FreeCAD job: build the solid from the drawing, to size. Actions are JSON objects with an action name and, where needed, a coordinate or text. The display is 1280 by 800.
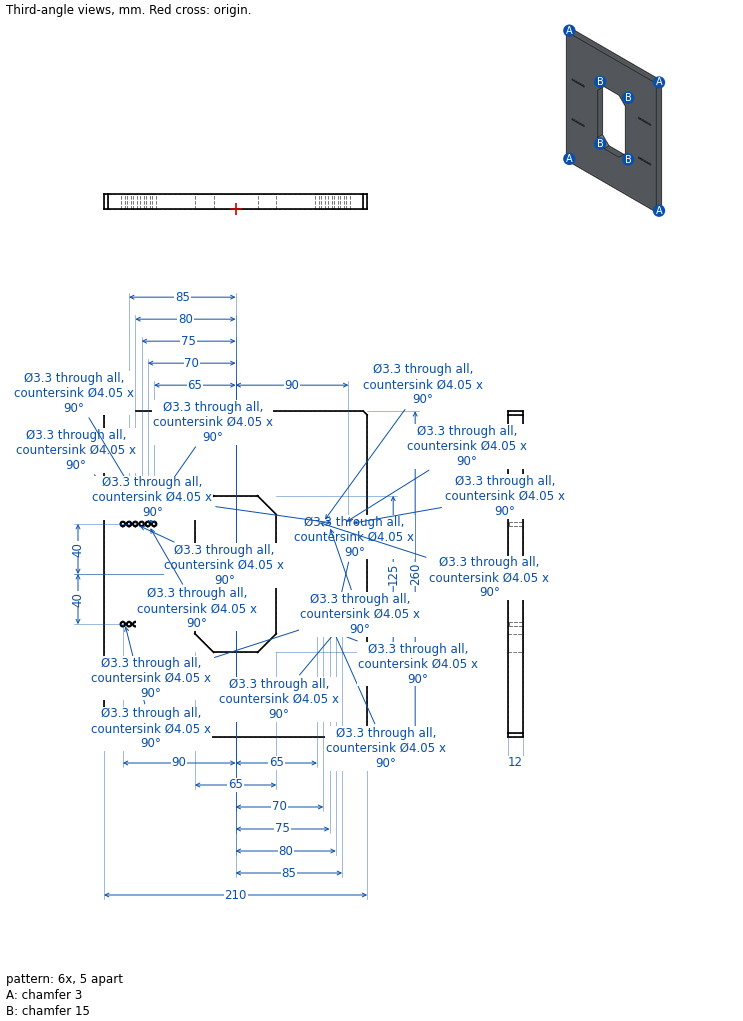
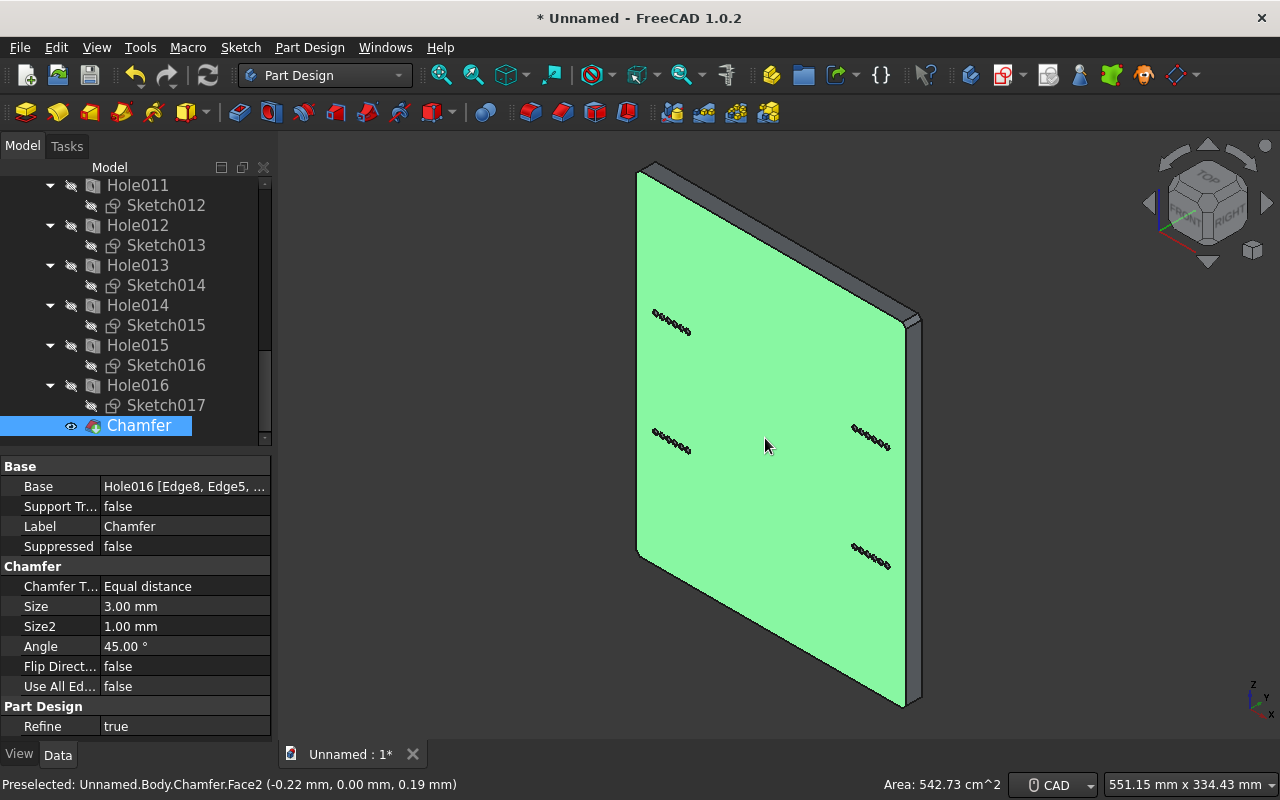
{"action": "left_click", "coordinate": [1004, 76]}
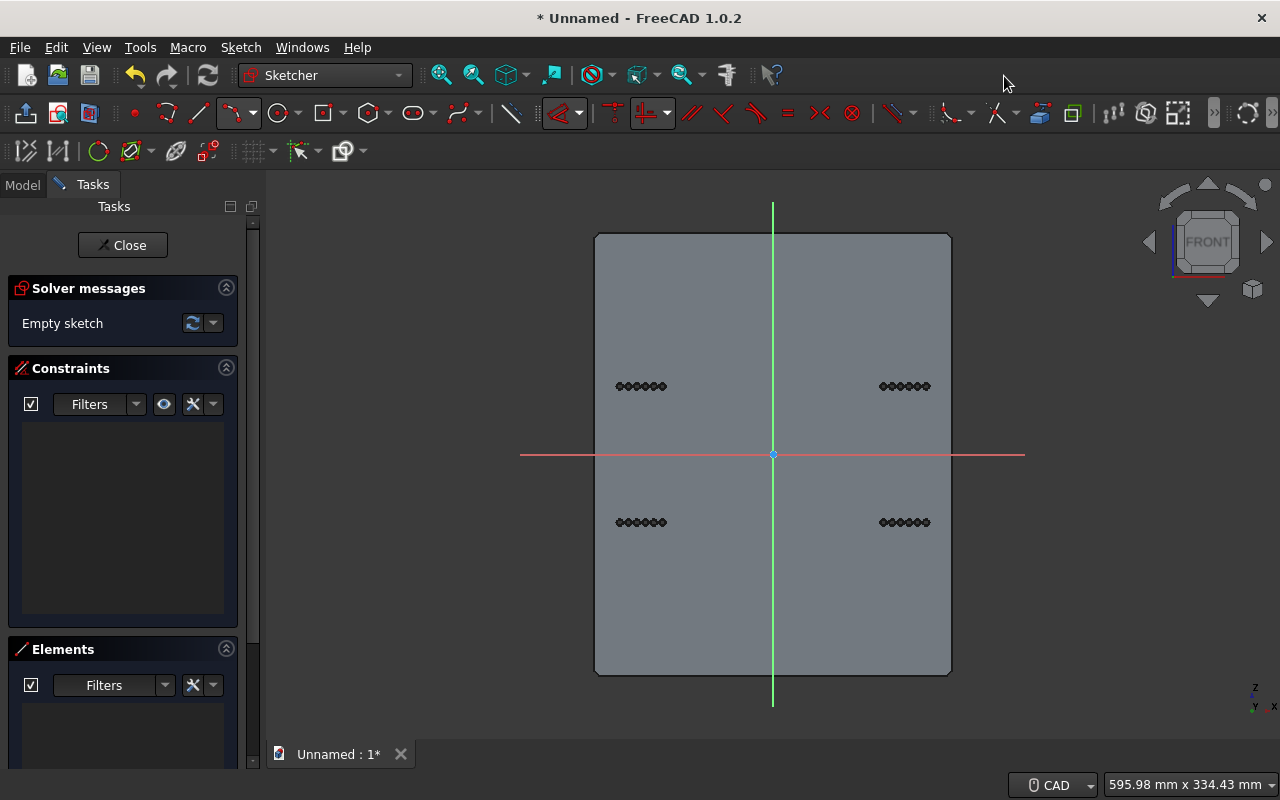
{"action": "scroll", "coordinate": [856, 455], "scroll_direction": "up", "scroll_amount": 3}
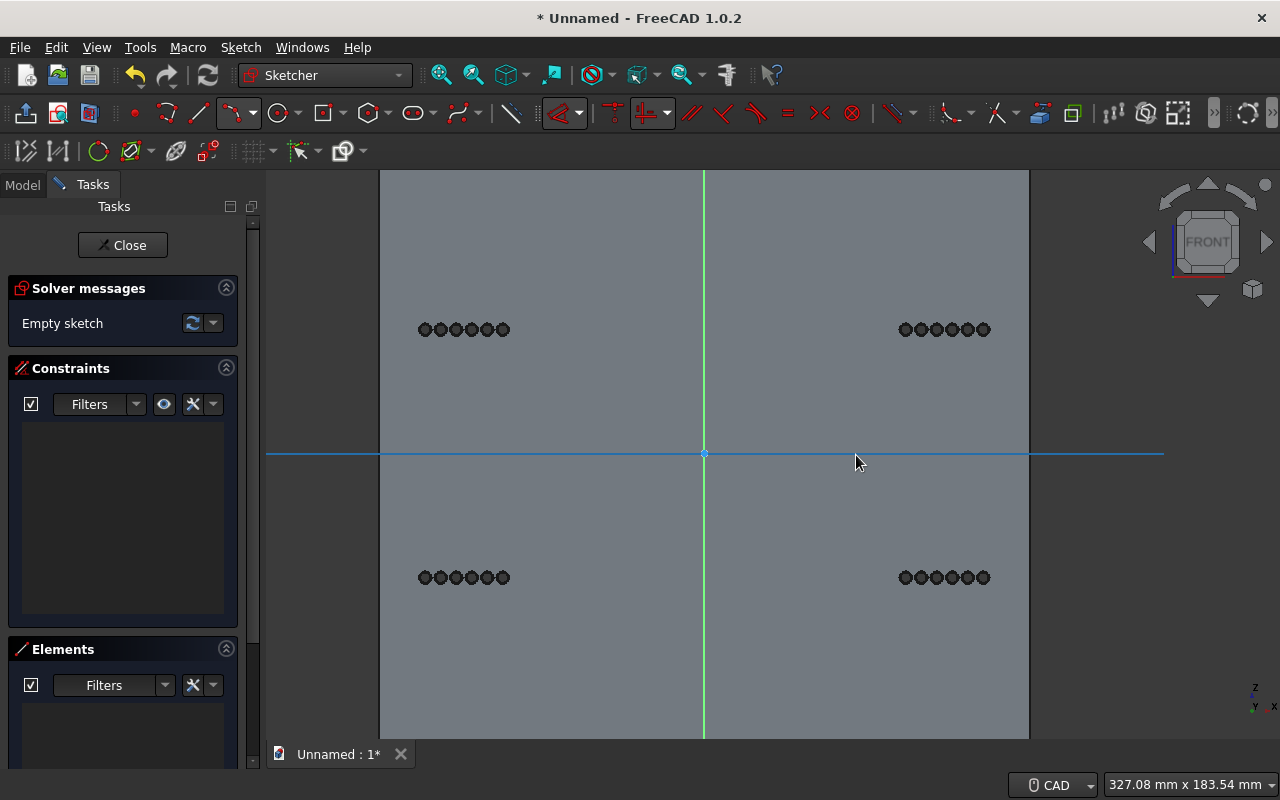
{"action": "left_click", "coordinate": [324, 114]}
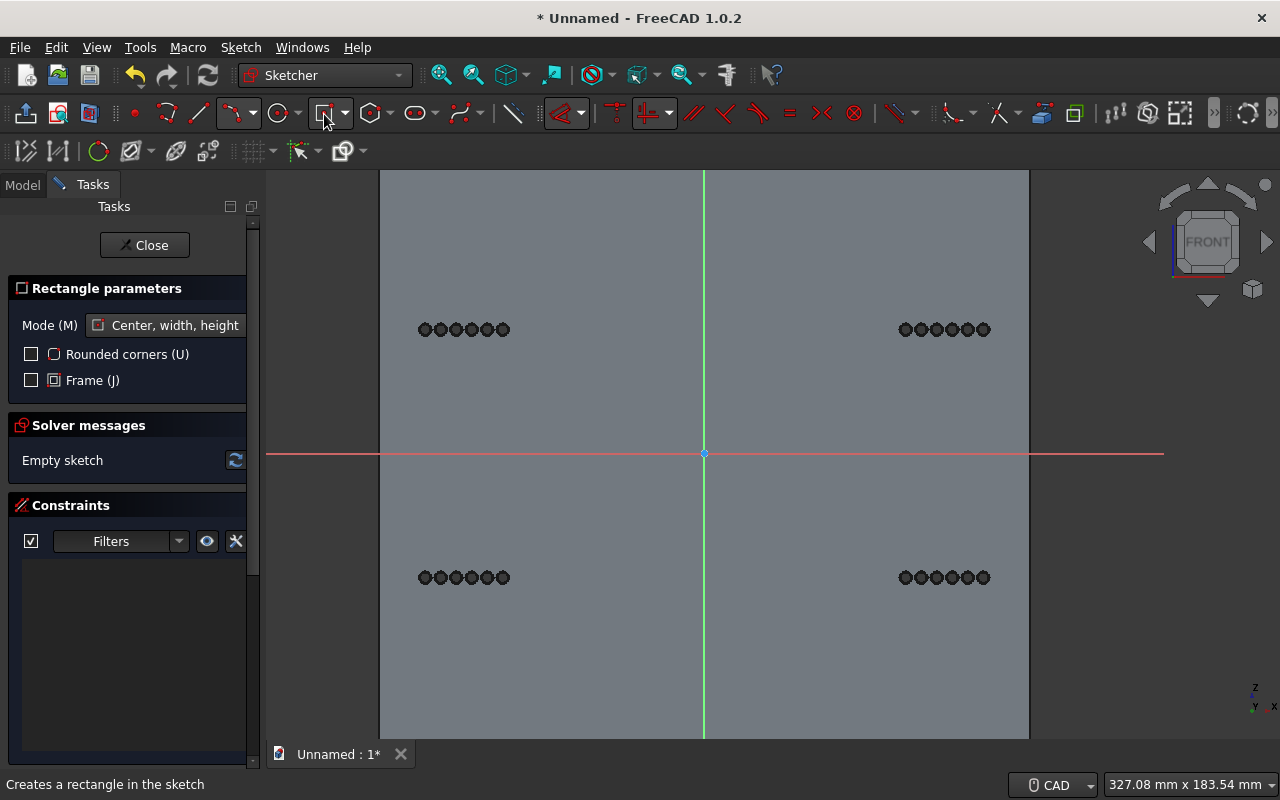
{"action": "left_click", "coordinate": [704, 454]}
{"action": "mouse_move", "coordinate": [805, 260]}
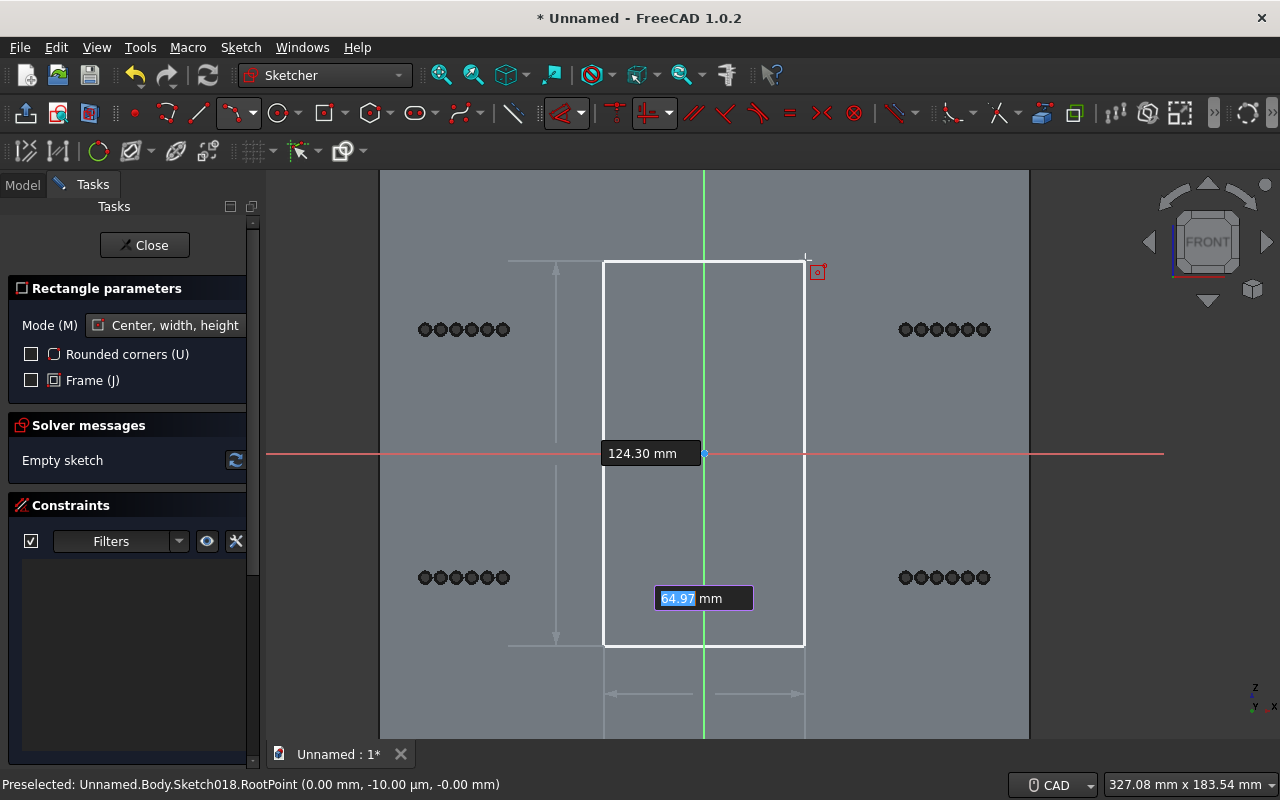
{"action": "type", "text": "65"}
{"action": "key", "text": "Tab"}
{"action": "type", "text": "125"}
{"action": "key", "text": "Return"}
{"action": "key", "text": "Escape"}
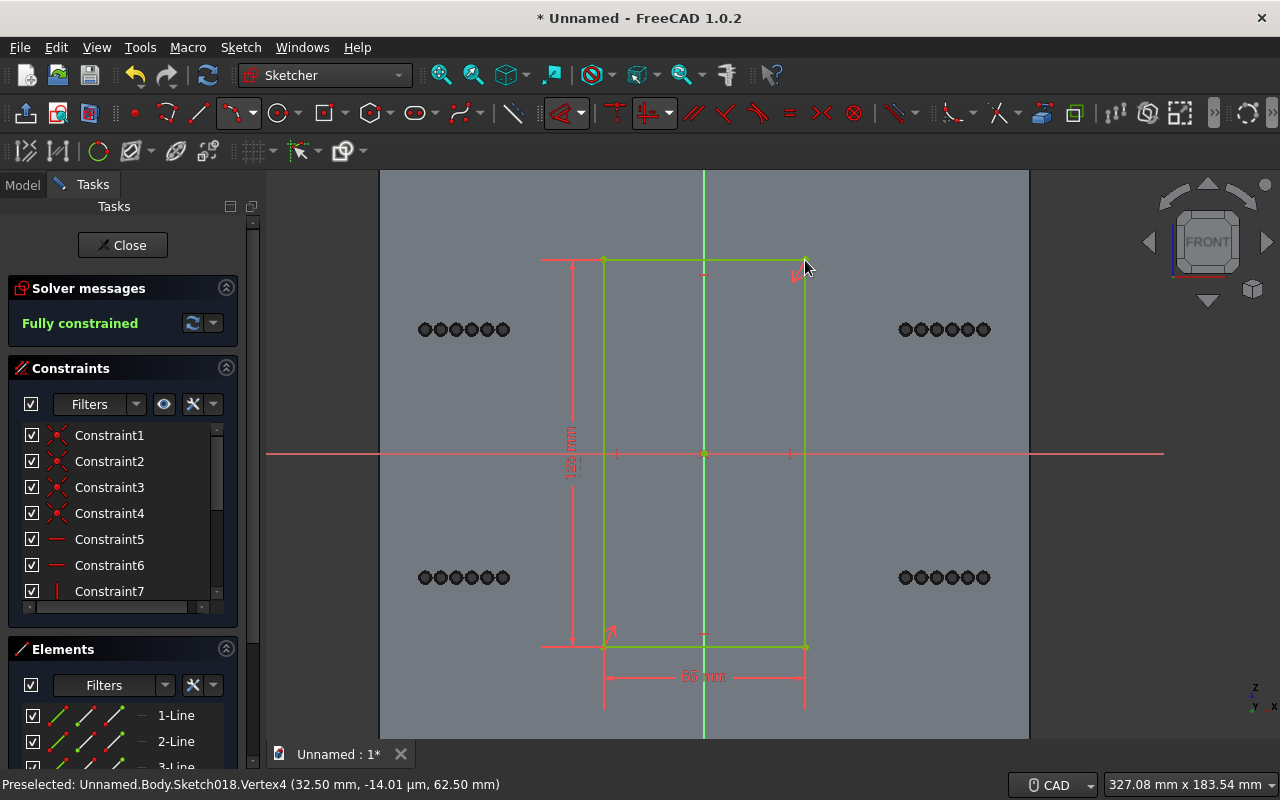
{"action": "left_click", "coordinate": [123, 245]}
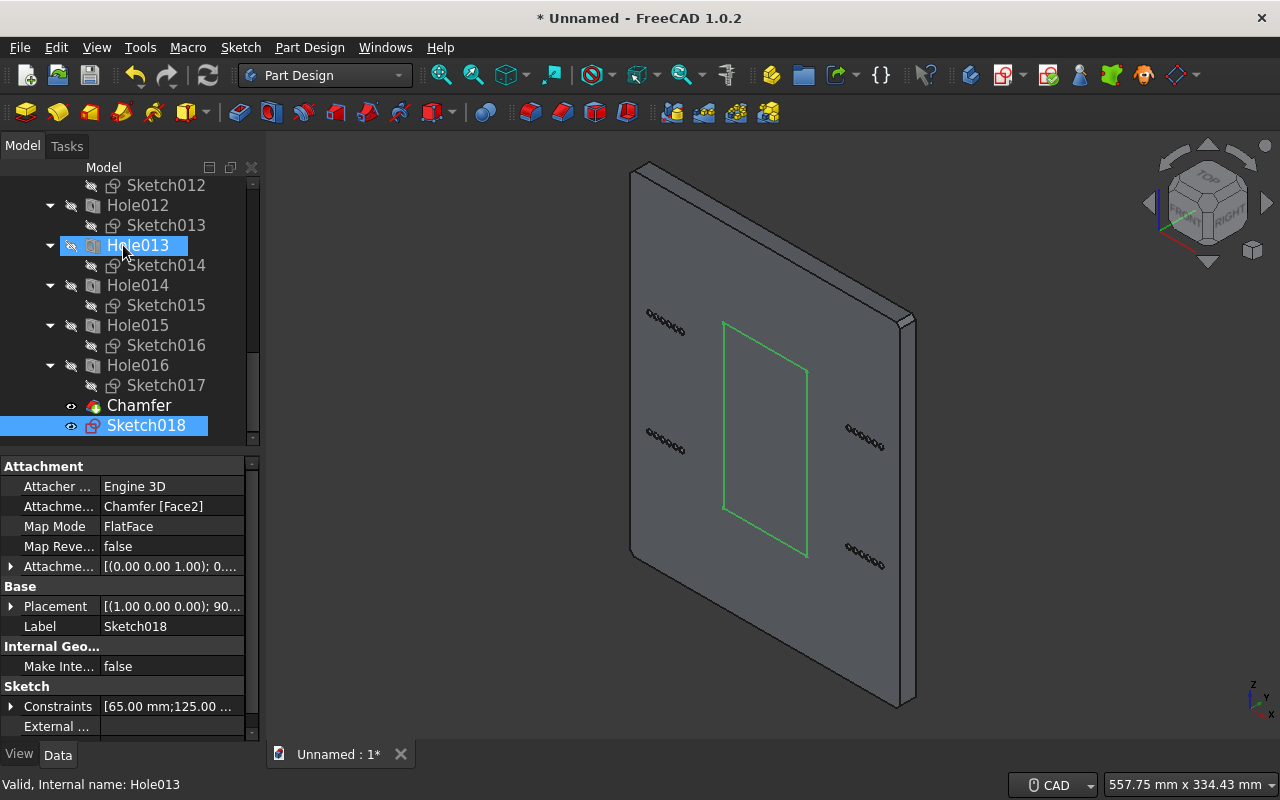
{"action": "left_click", "coordinate": [240, 112]}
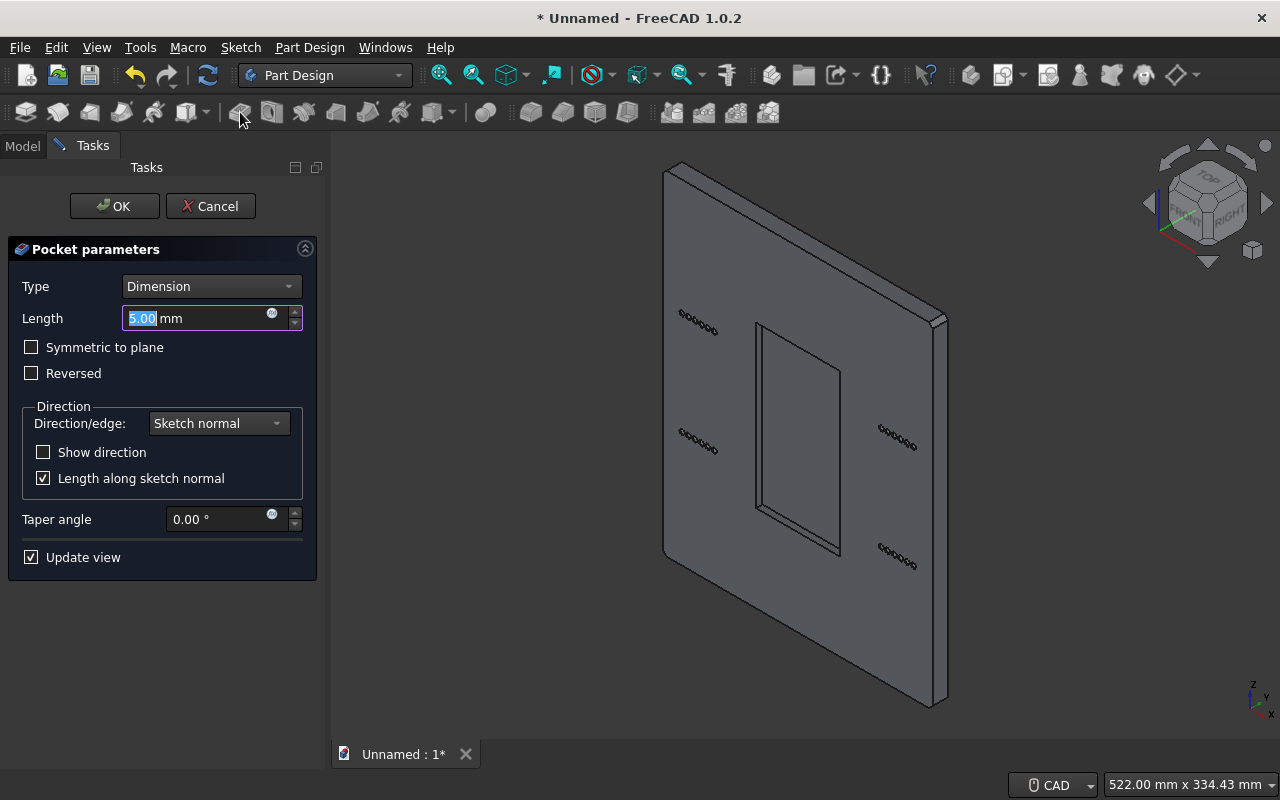
{"action": "left_click", "coordinate": [212, 286]}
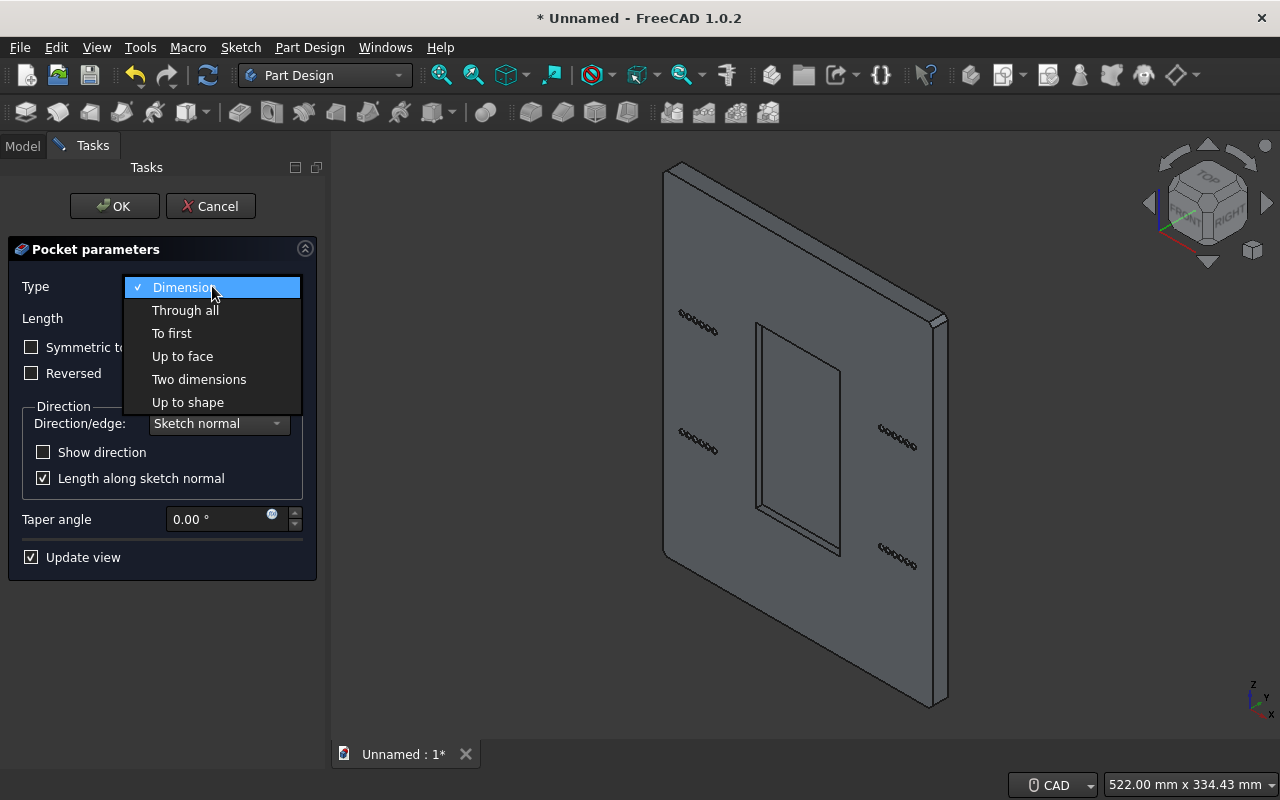
{"action": "left_click", "coordinate": [212, 334]}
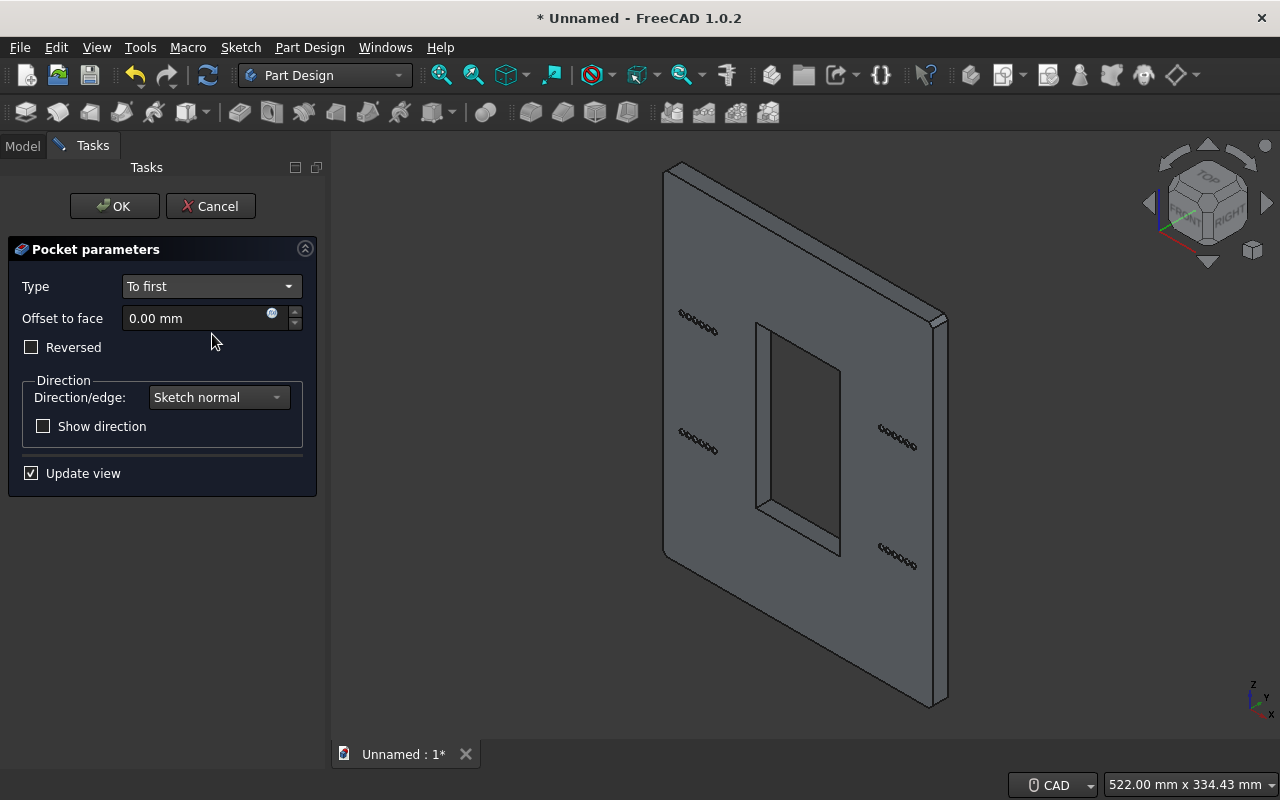
{"action": "left_click", "coordinate": [115, 206]}